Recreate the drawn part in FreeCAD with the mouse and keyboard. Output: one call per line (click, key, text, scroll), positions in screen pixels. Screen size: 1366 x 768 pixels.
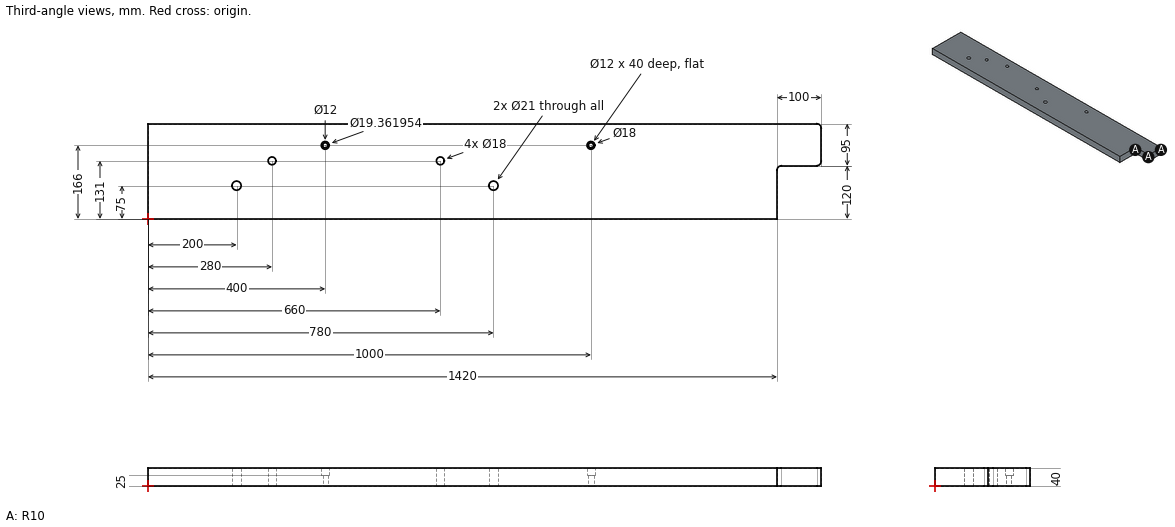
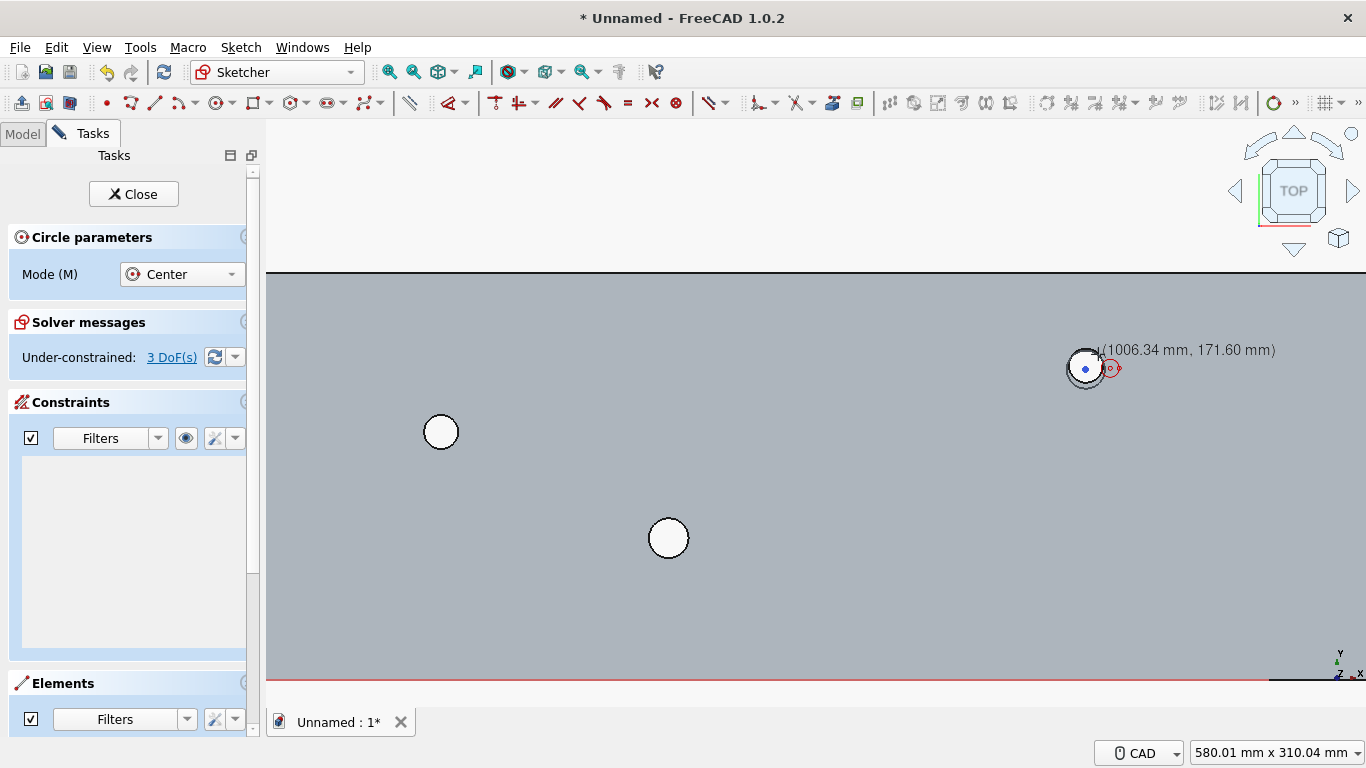
scroll(1097, 354, down, 5)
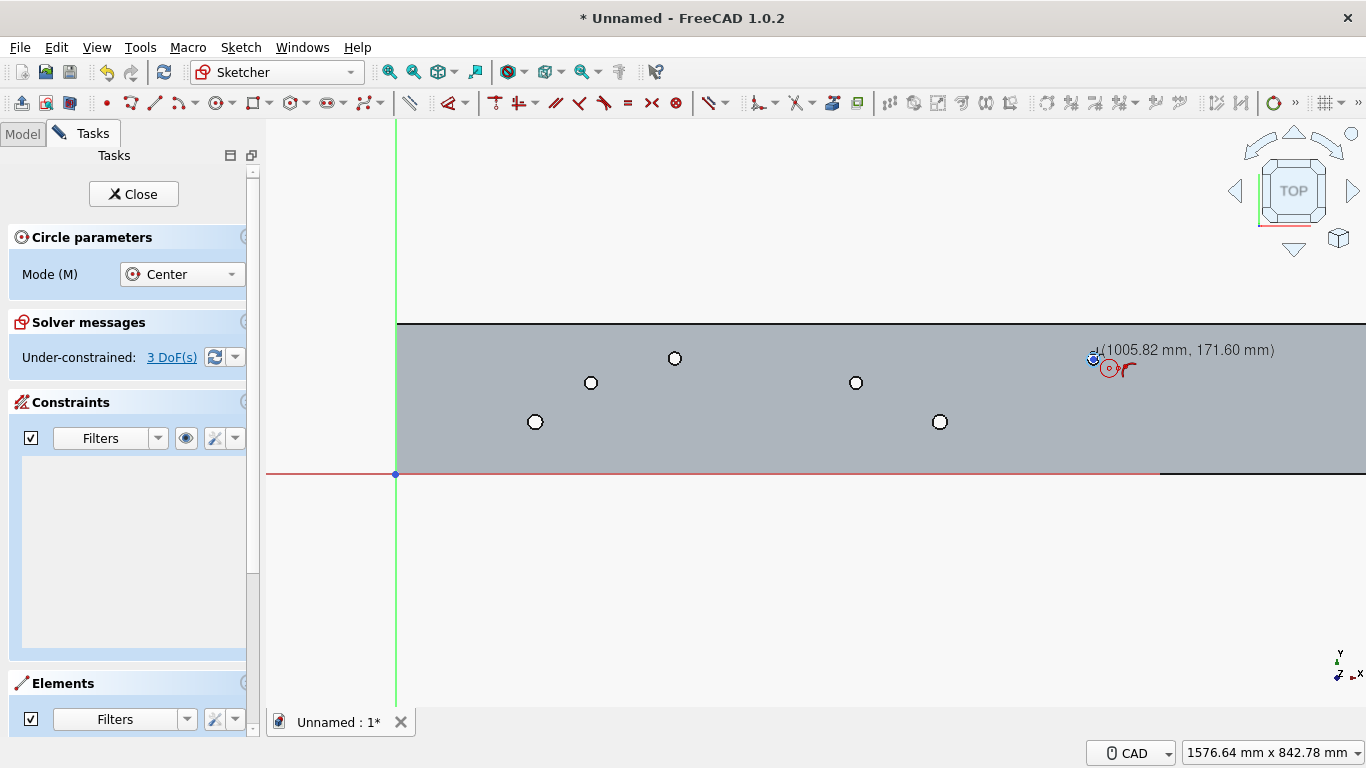
scroll(675, 359, up, 7)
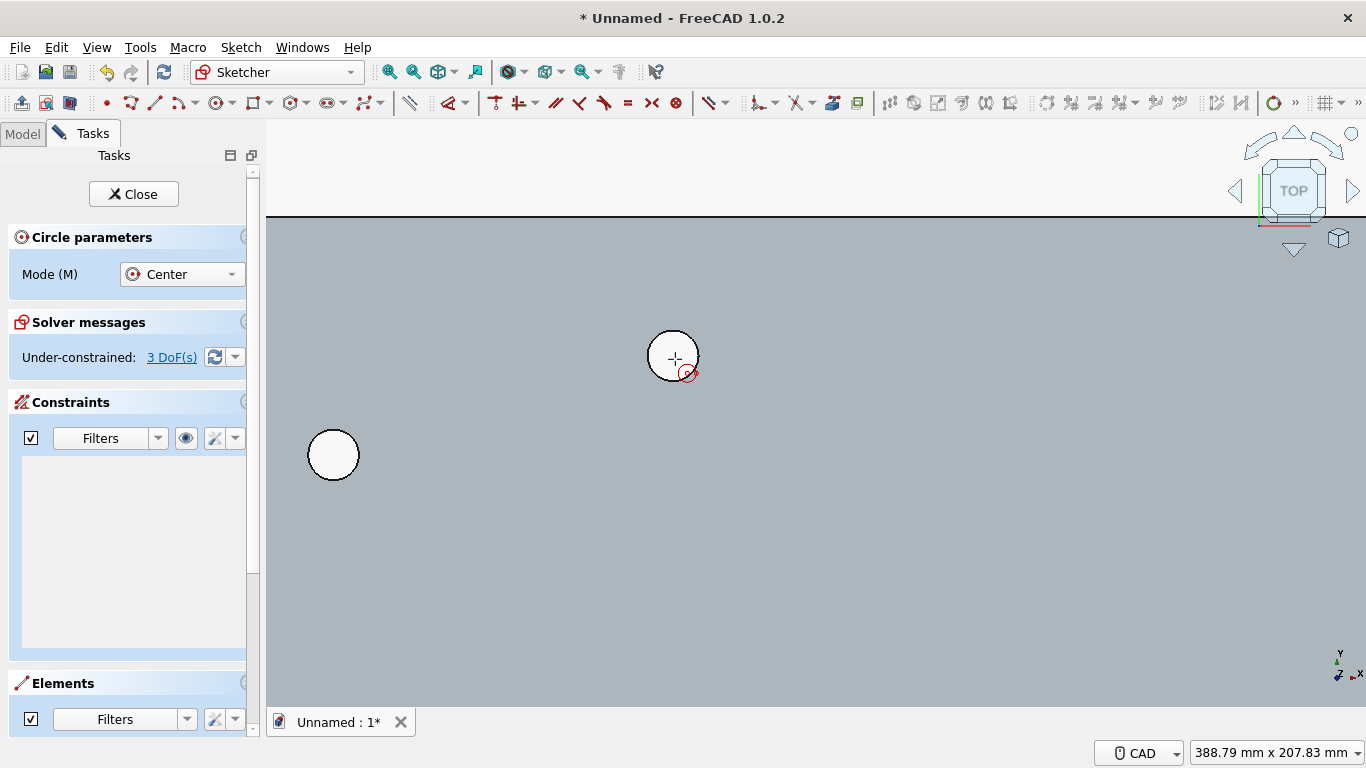
scroll(675, 359, down, 7)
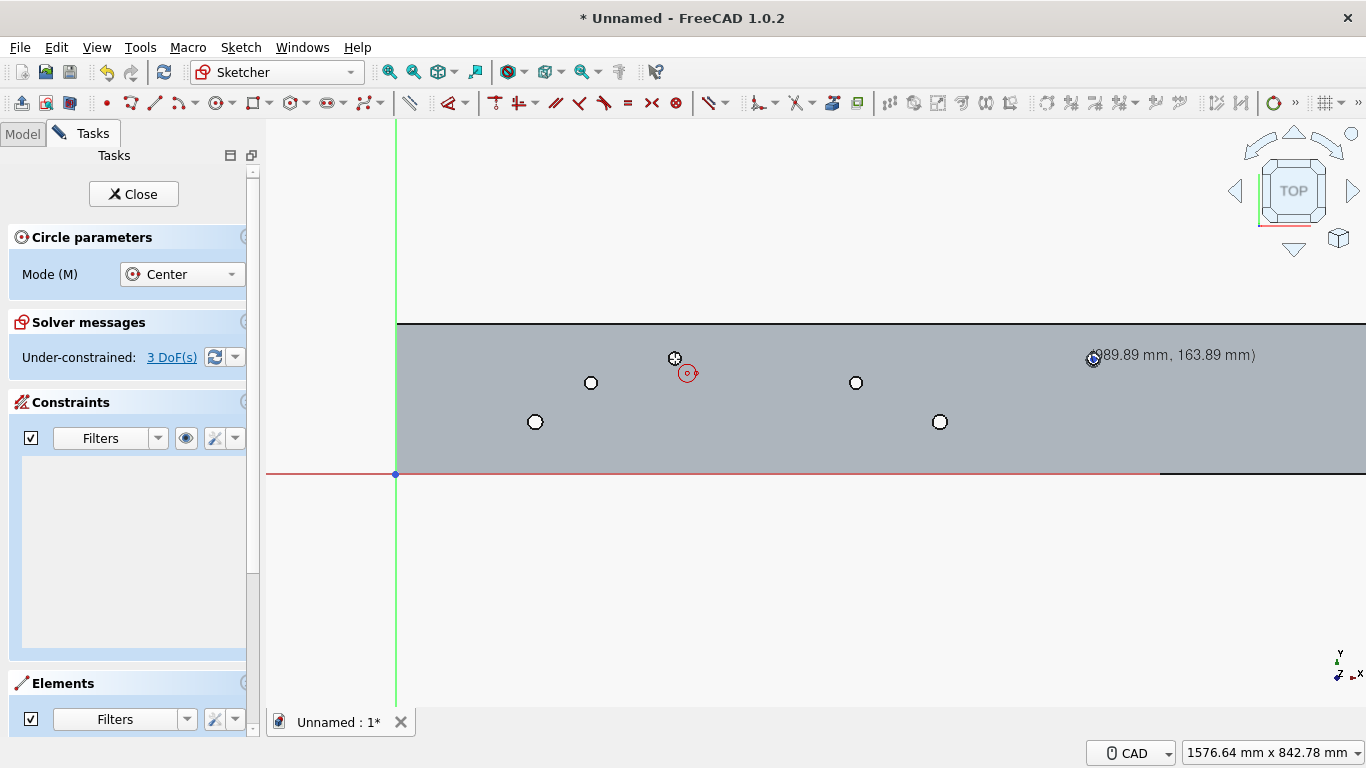
click(675, 359)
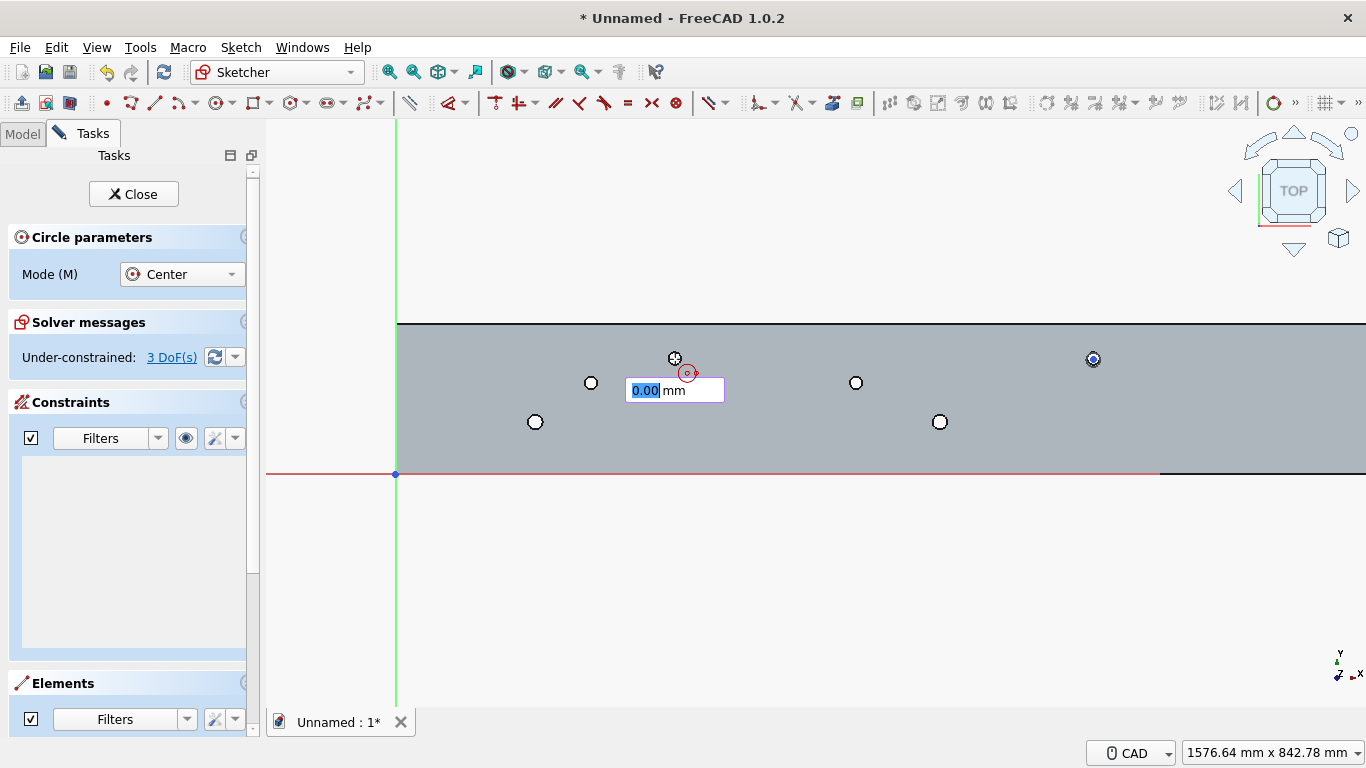
scroll(680, 354, up, 5)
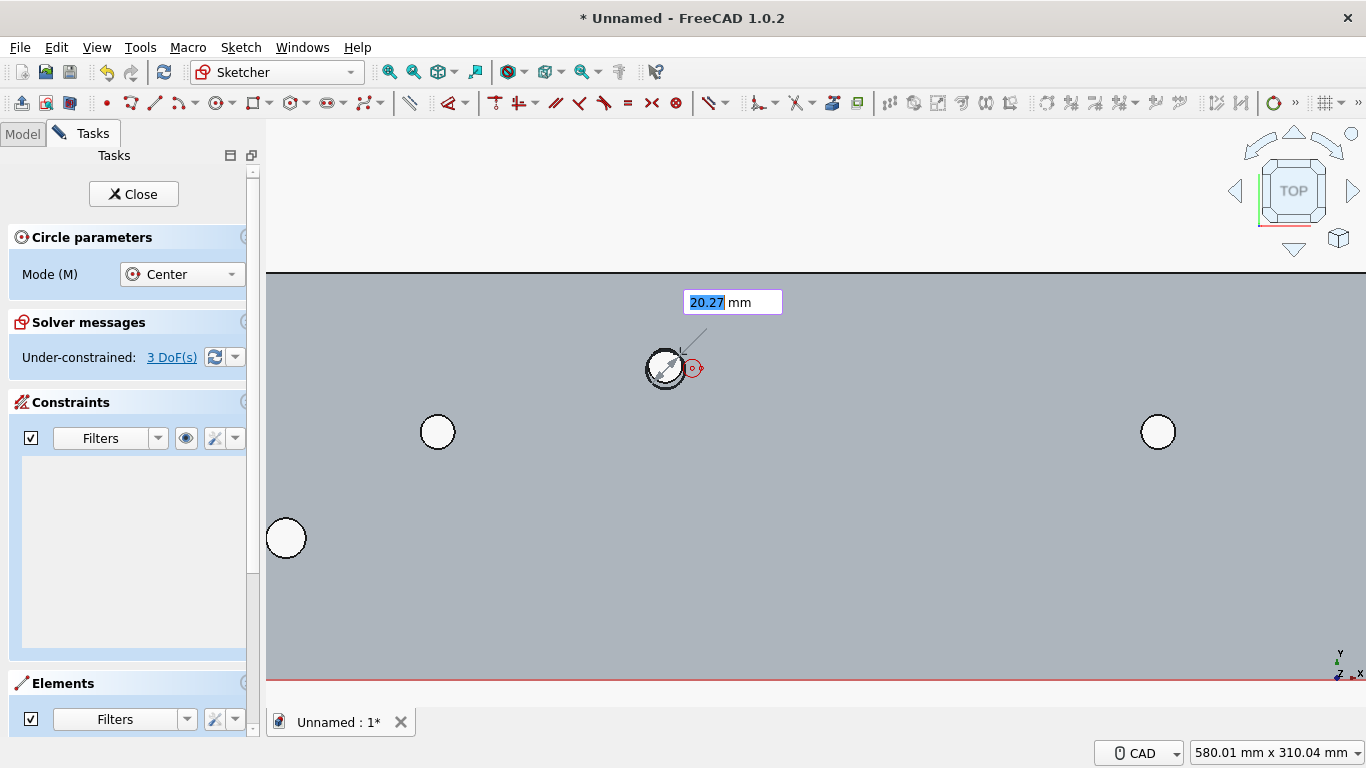
click(678, 353)
key(Escape)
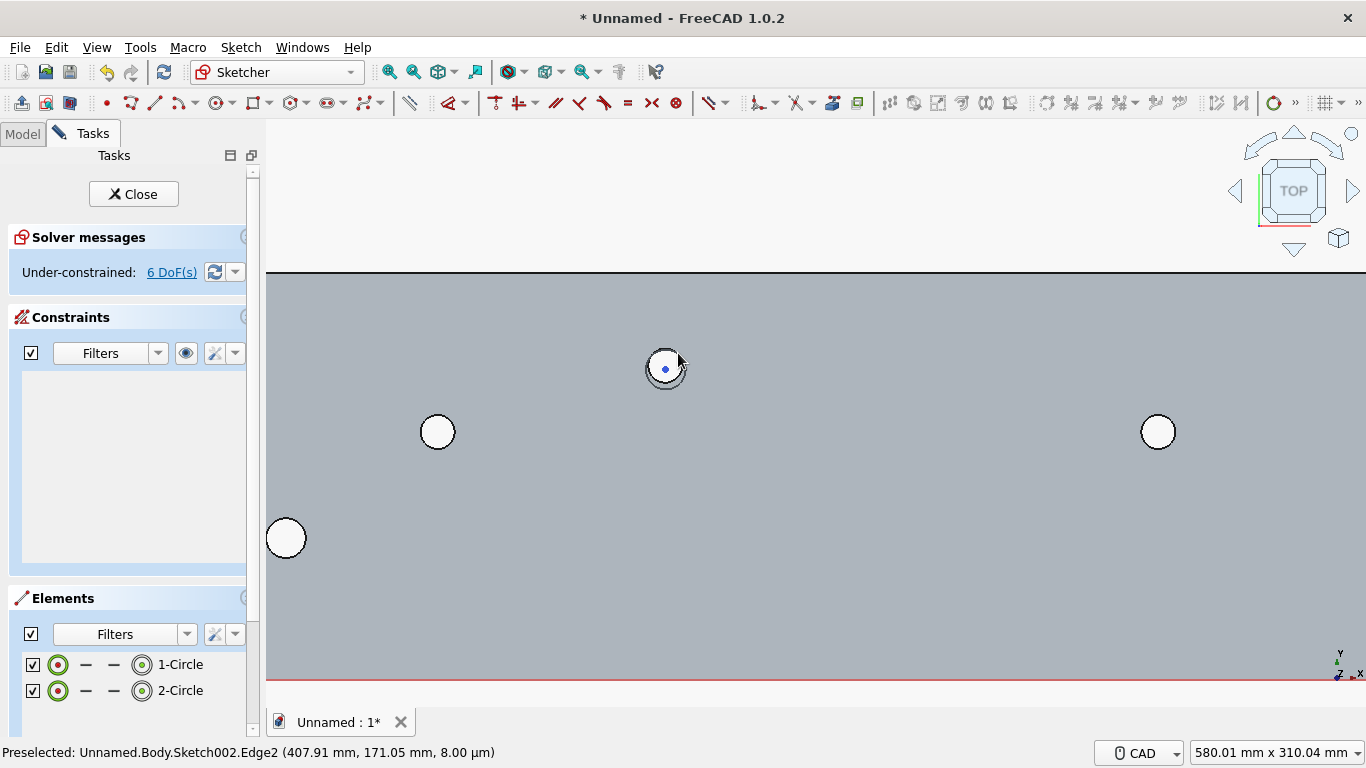
click(448, 104)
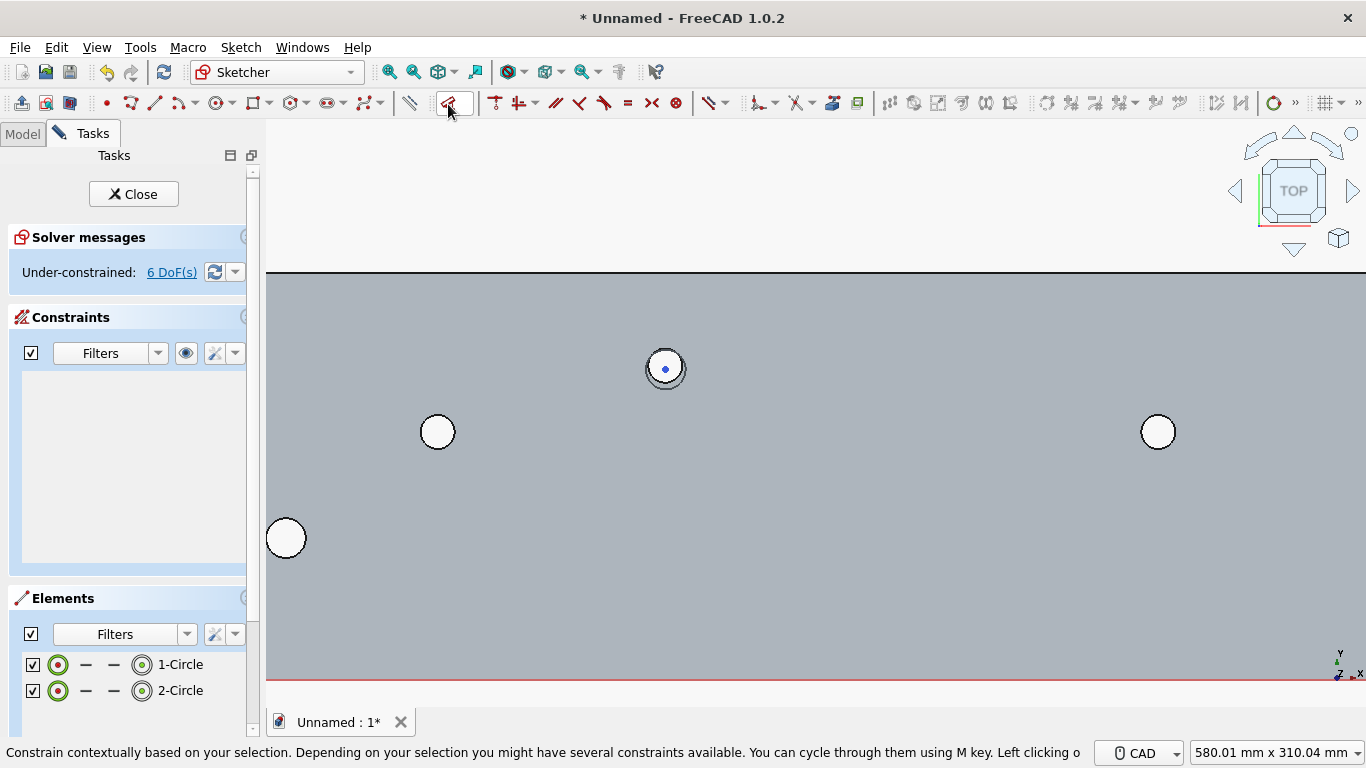
scroll(680, 354, down, 5)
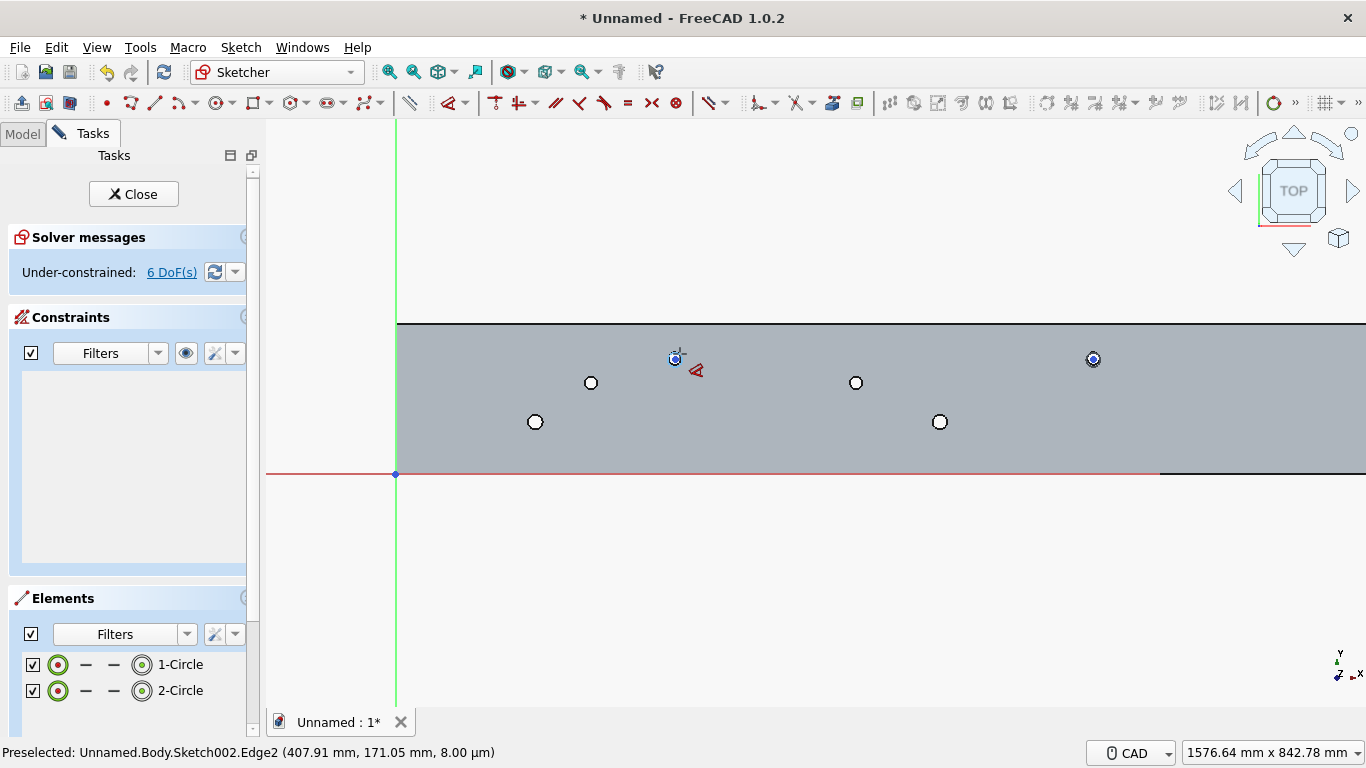
scroll(1098, 355, up, 6)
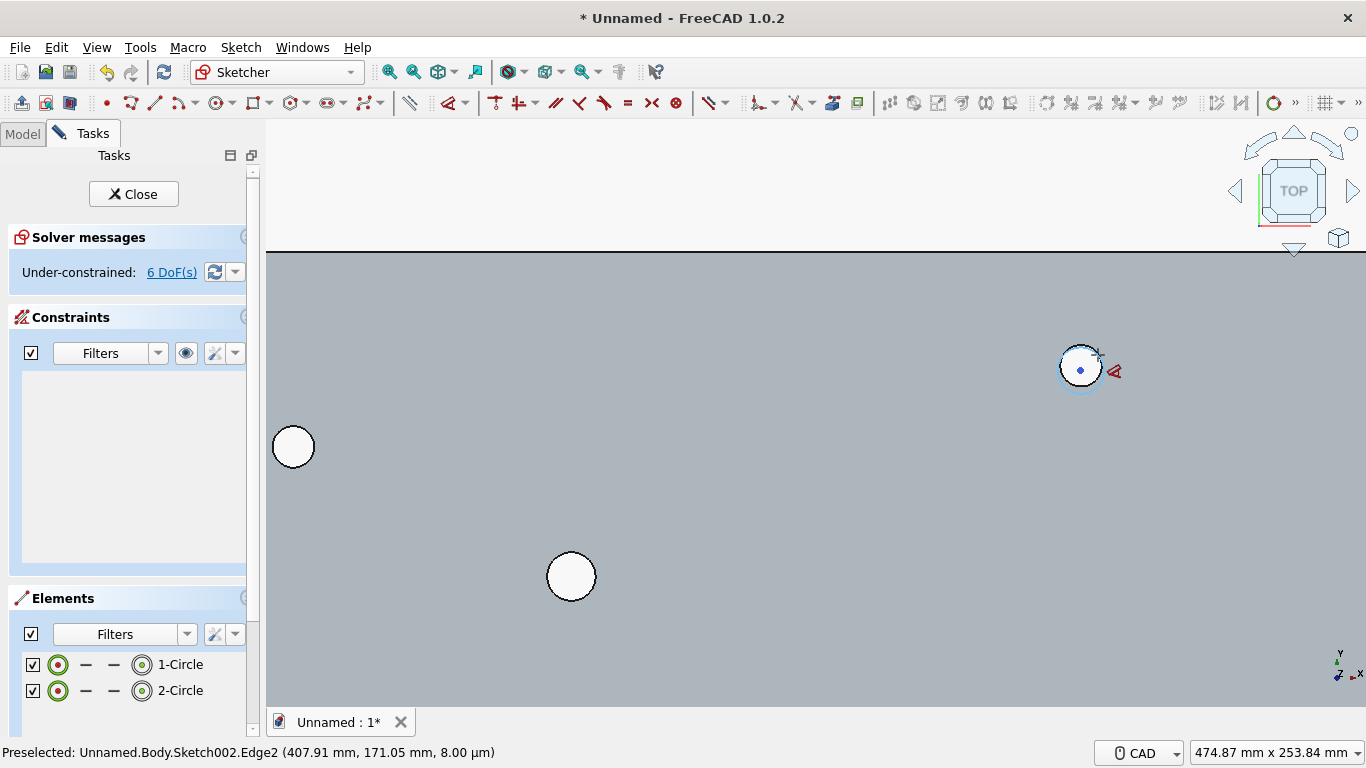
click(1097, 354)
click(1119, 331)